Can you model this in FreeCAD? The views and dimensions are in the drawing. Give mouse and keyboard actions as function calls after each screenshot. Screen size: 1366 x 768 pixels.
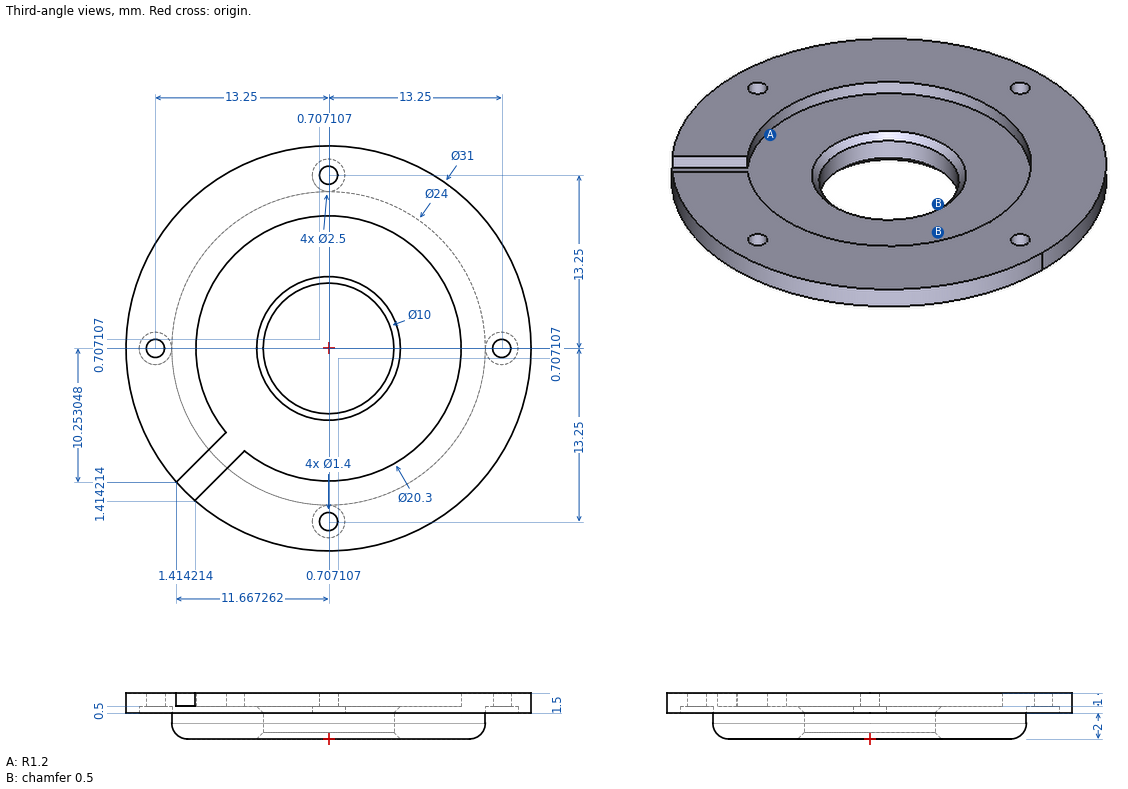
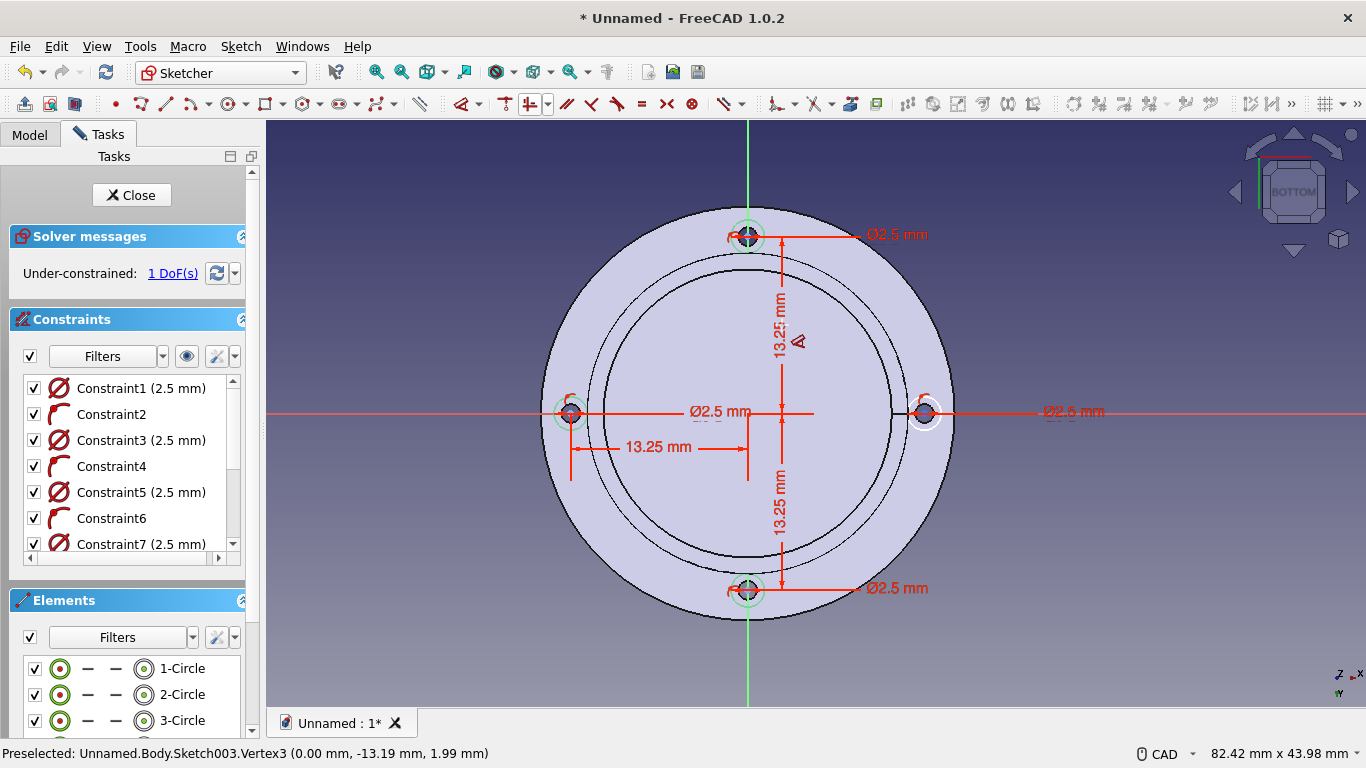
click(924, 414)
click(836, 448)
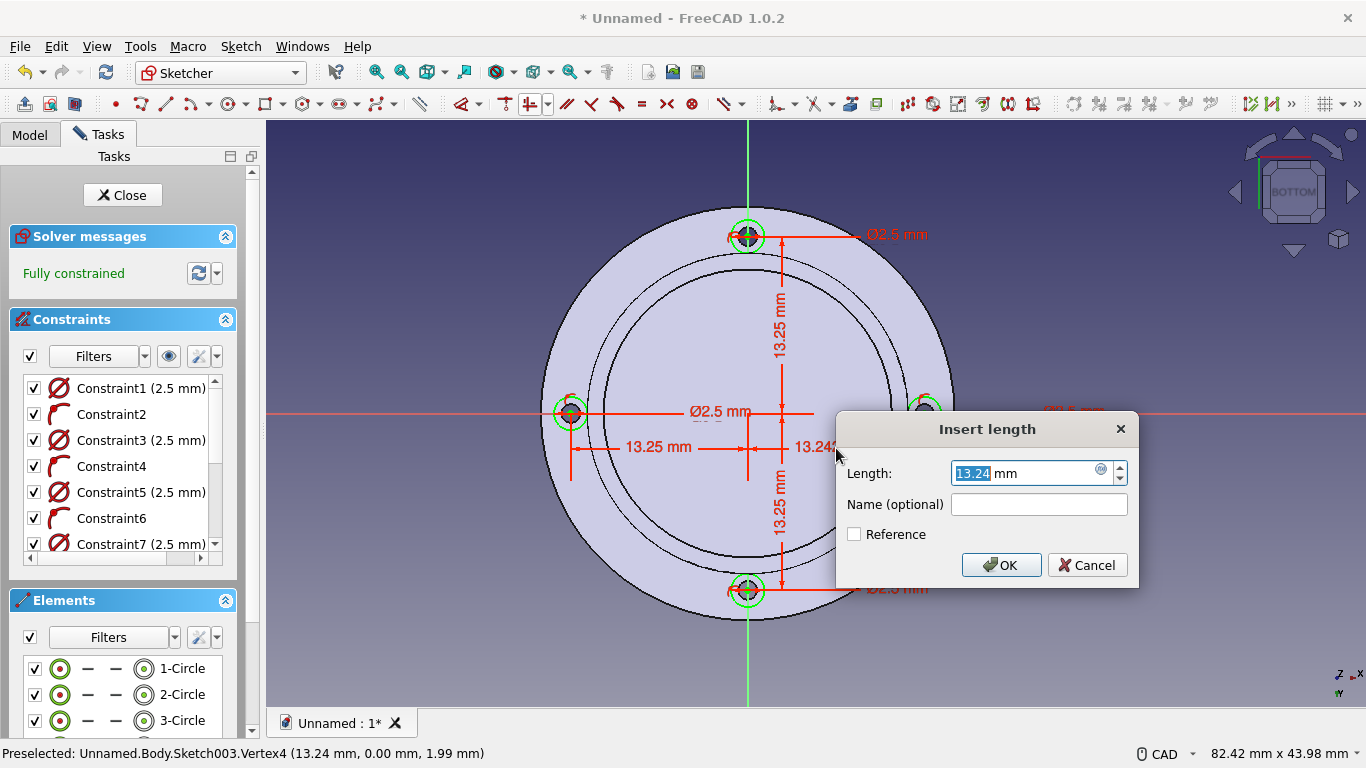
text(13.25)
key(Return)
key(Escape)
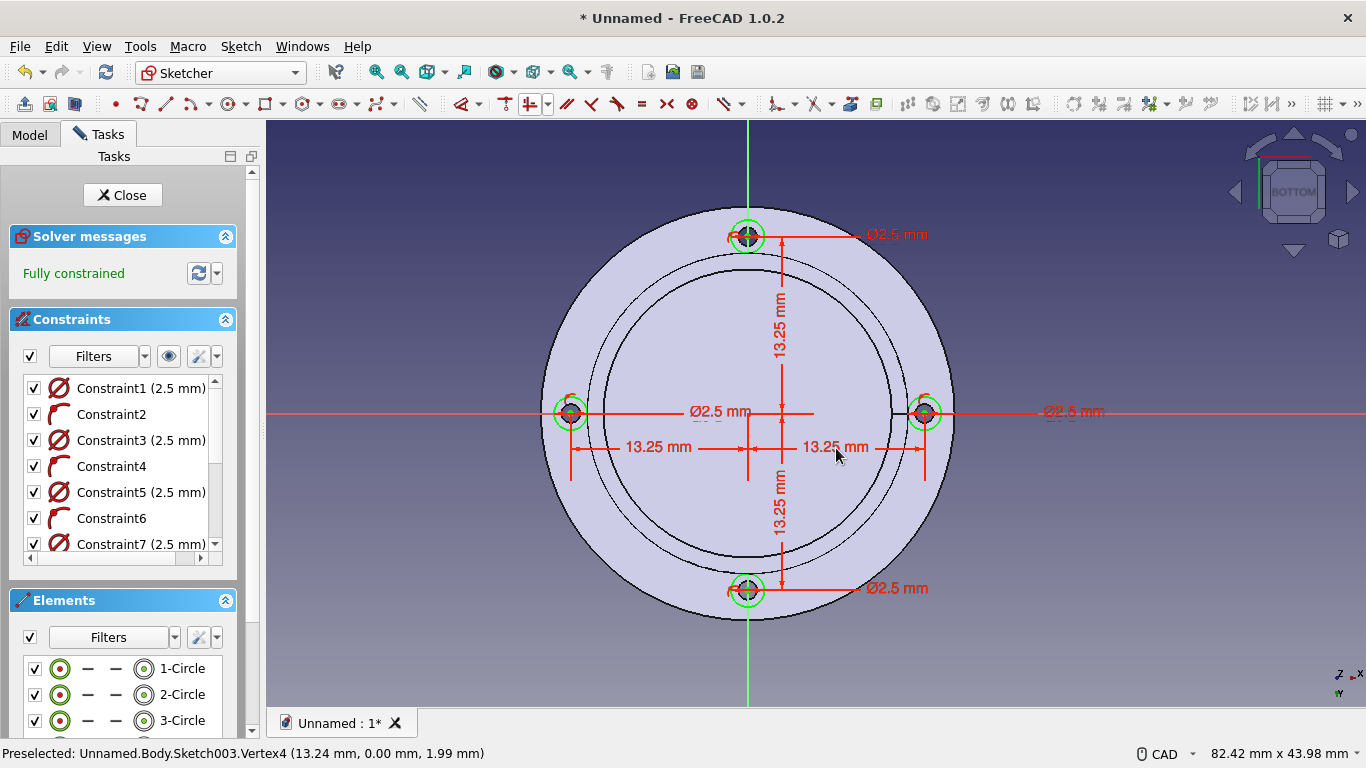
click(123, 195)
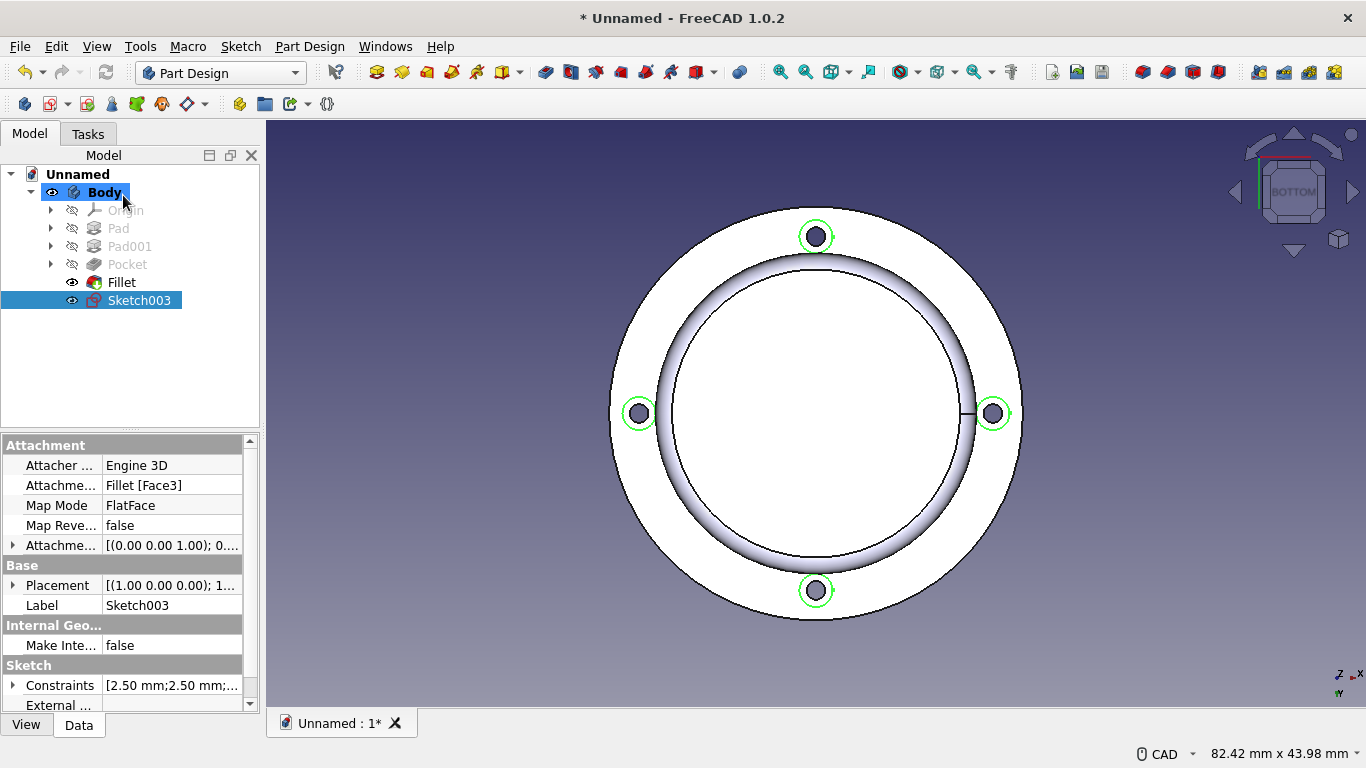
click(546, 72)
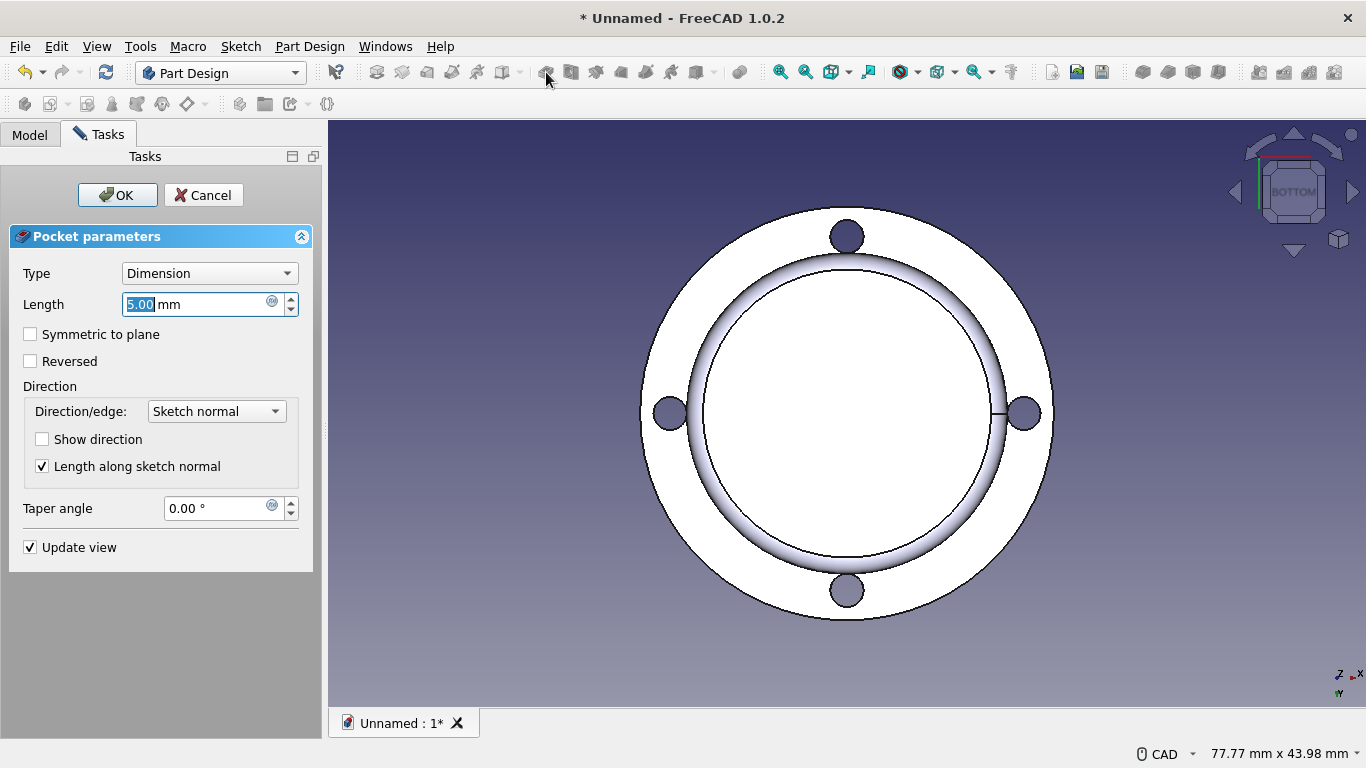
text(0.5)
key(Tab)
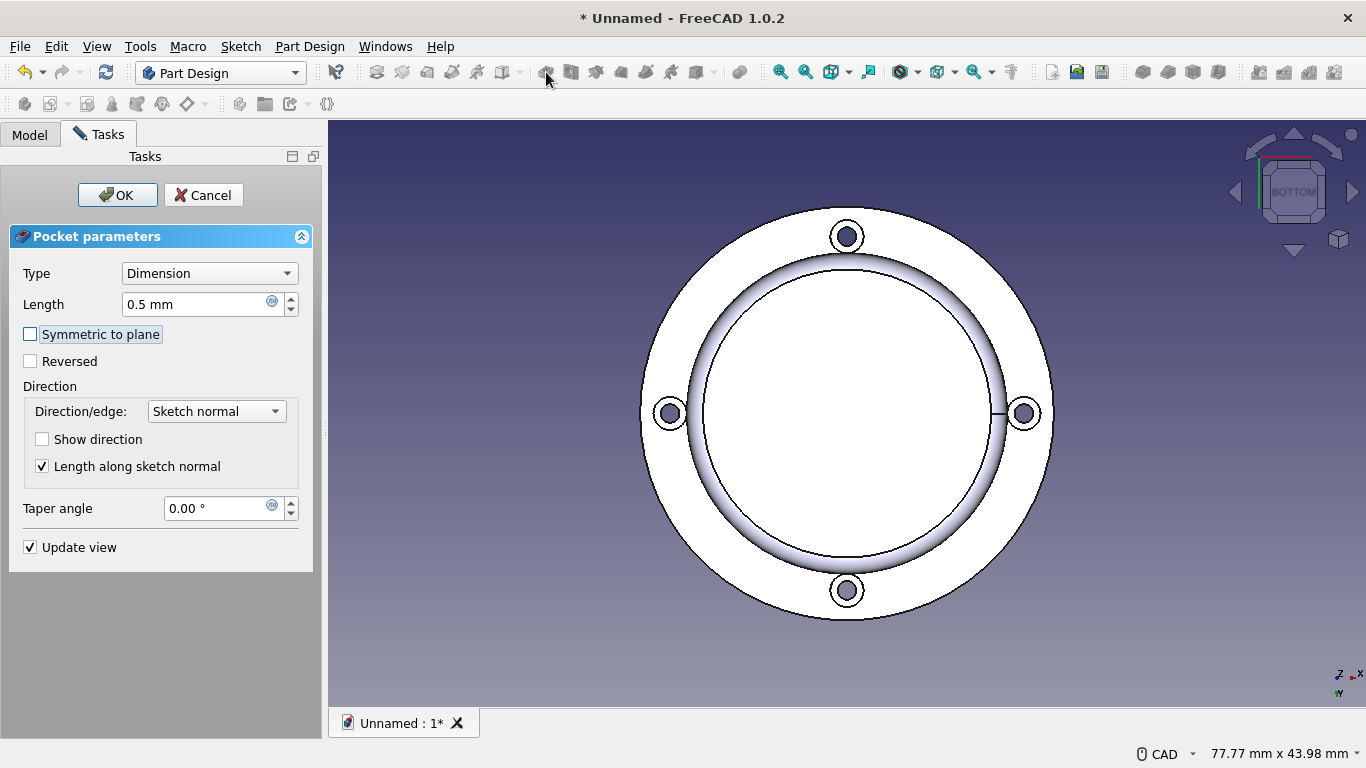
click(118, 195)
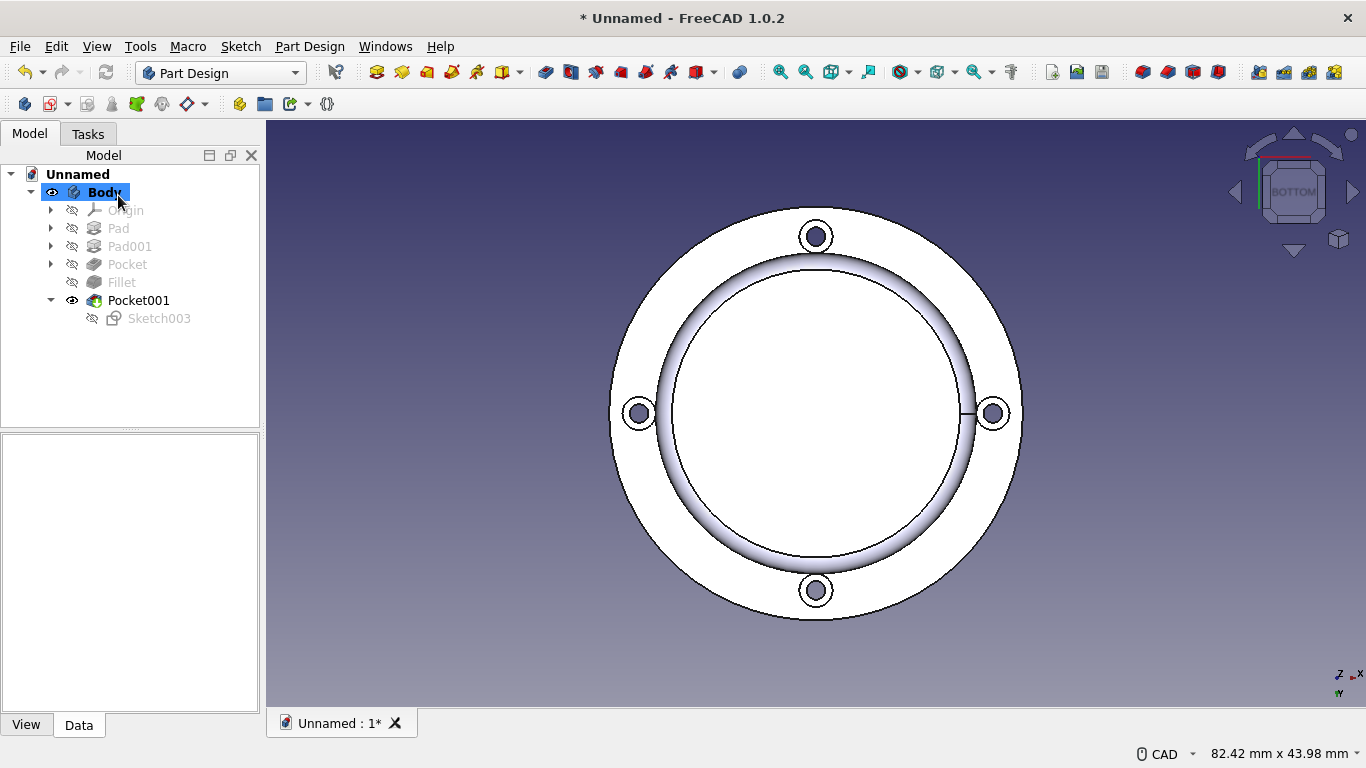
click(816, 413)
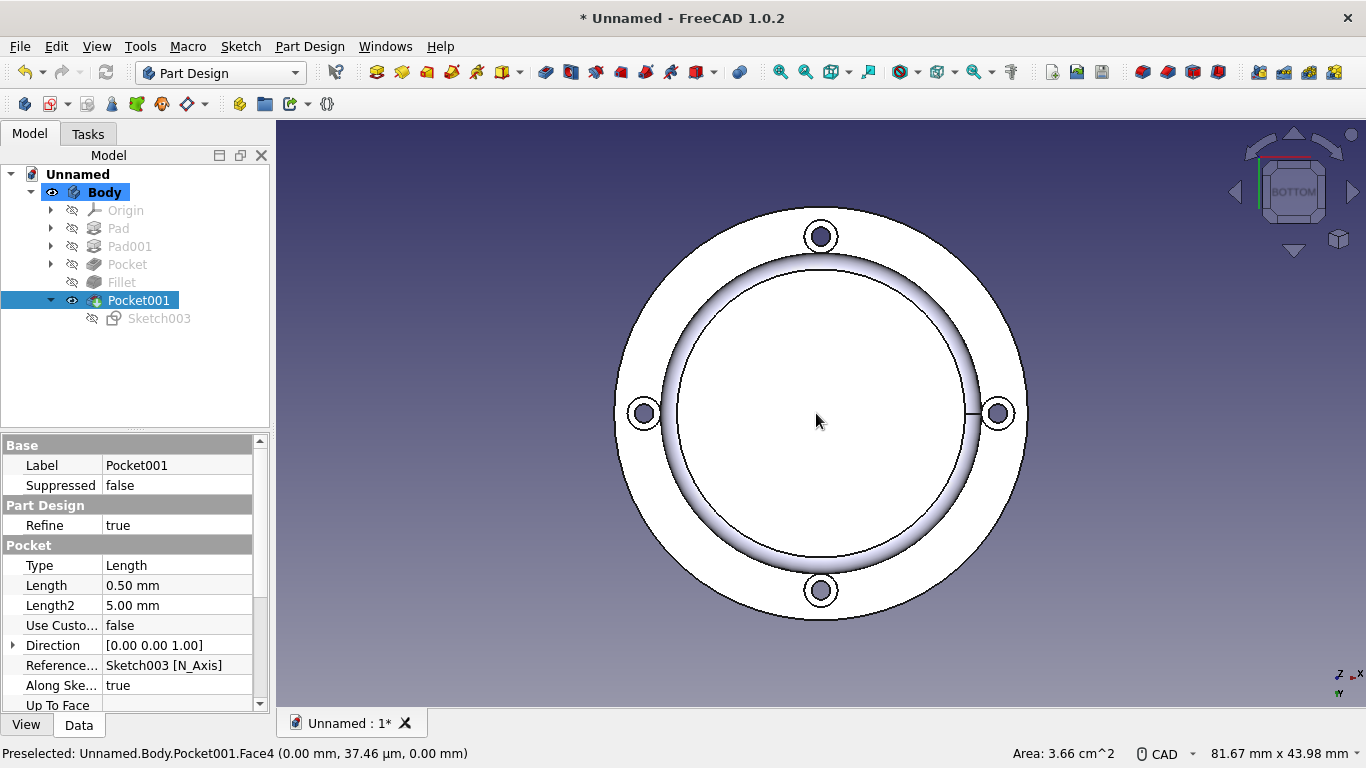
click(50, 104)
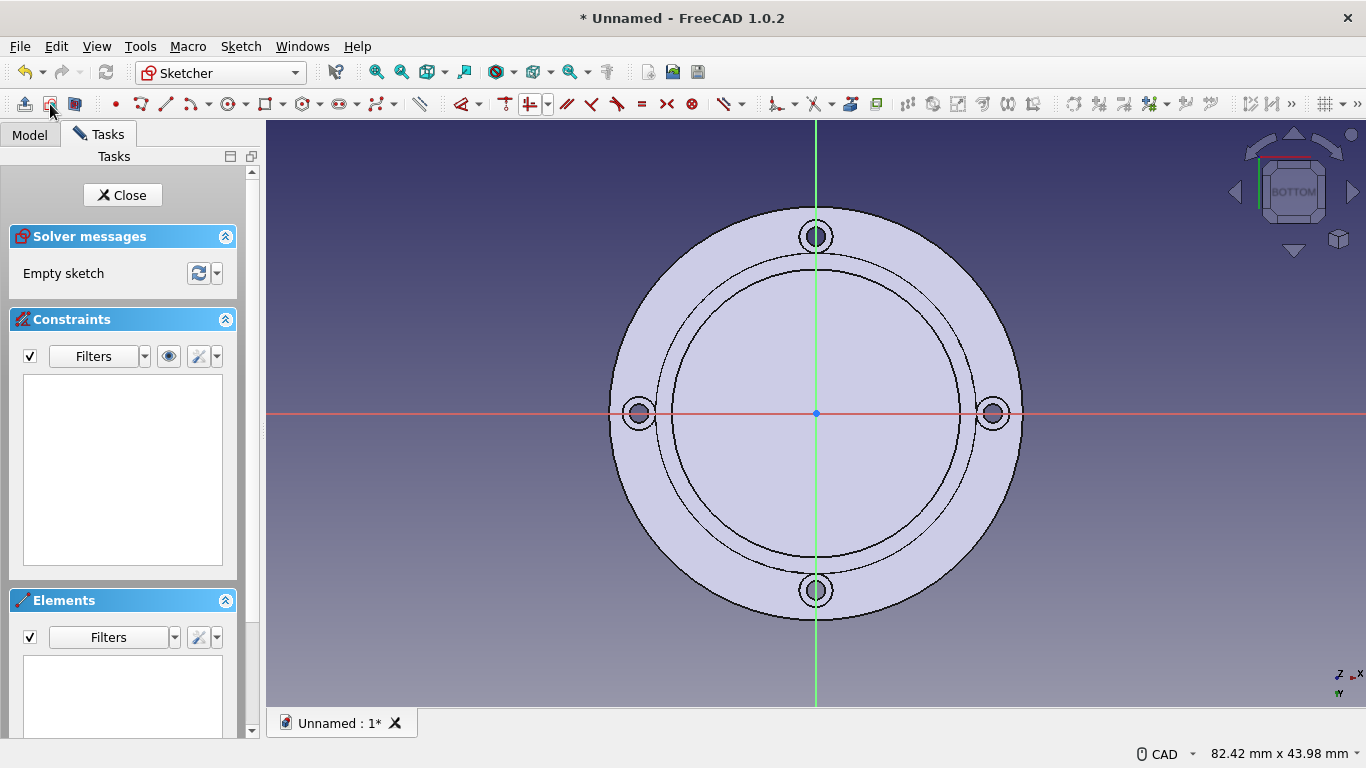
scroll(856, 414, up, 5)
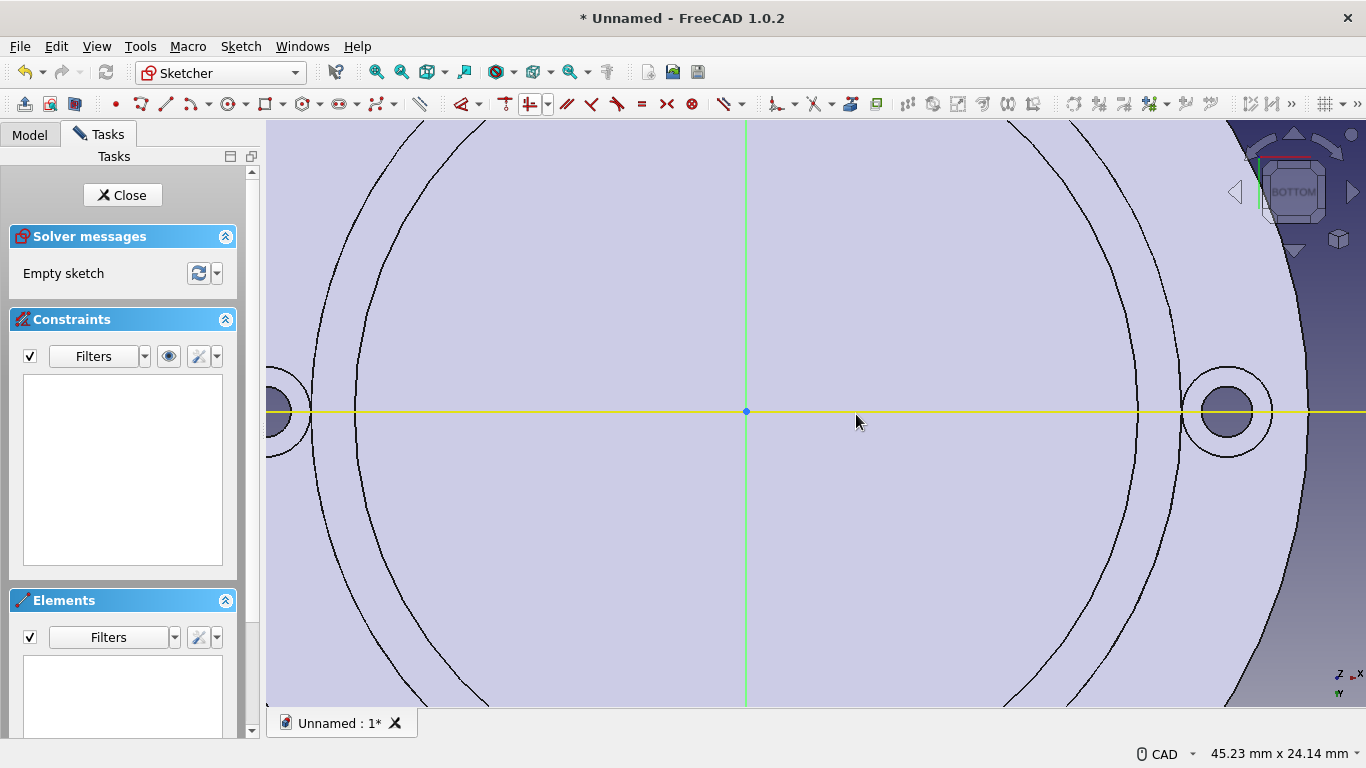
key(g)
key(c)